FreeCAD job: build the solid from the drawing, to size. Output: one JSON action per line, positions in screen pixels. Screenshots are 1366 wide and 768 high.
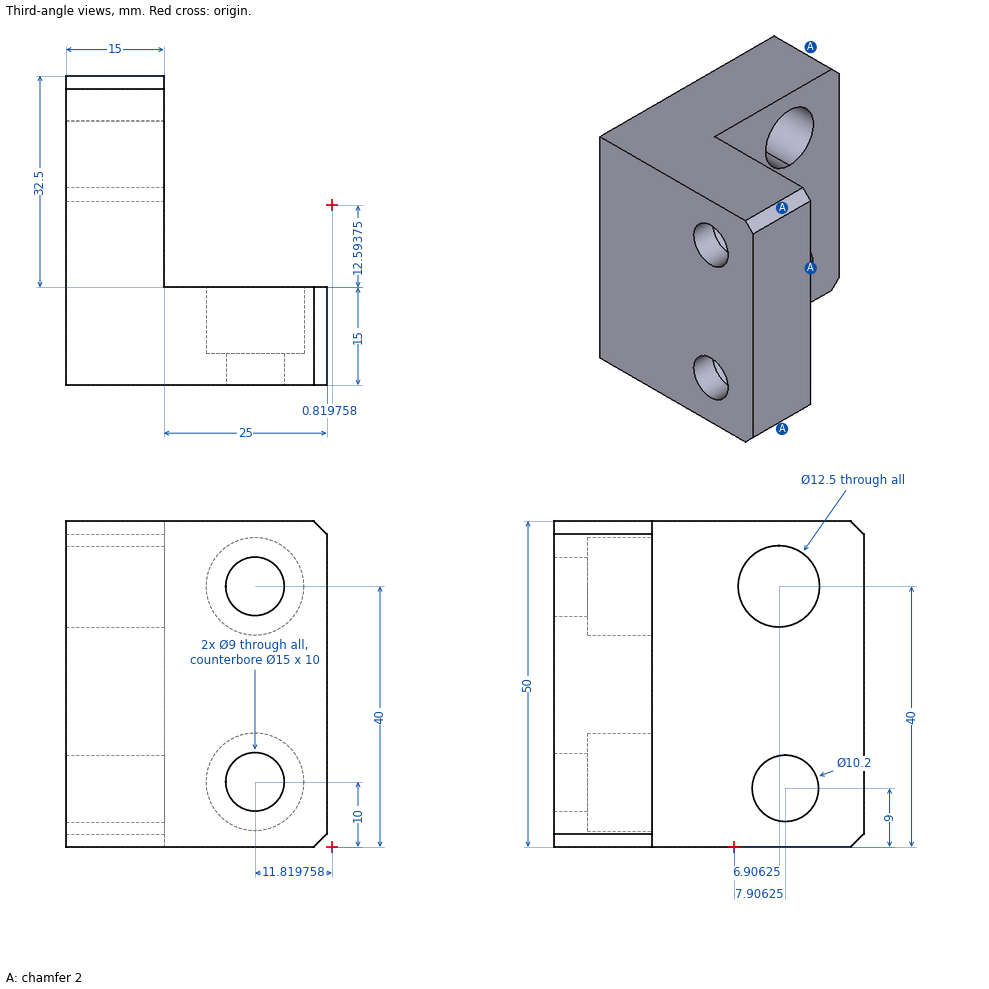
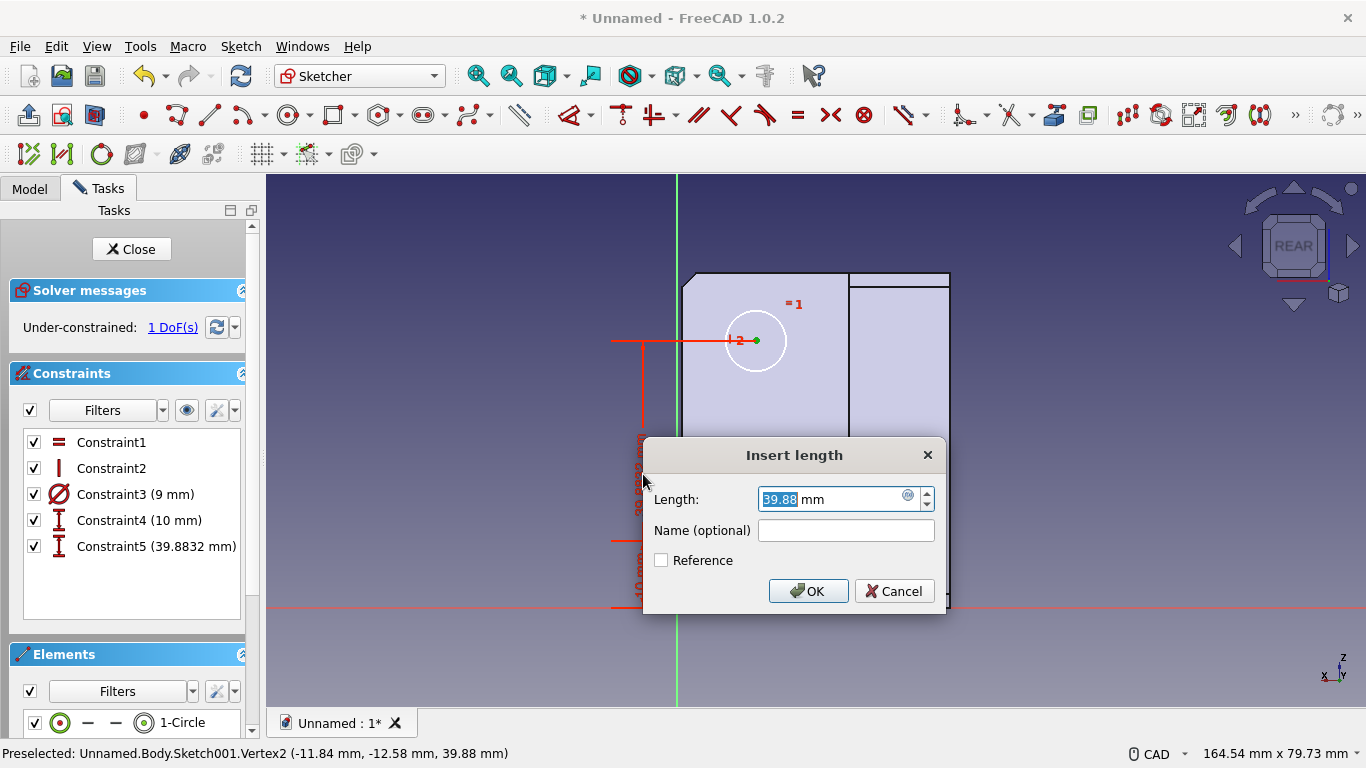
{"action": "type", "text": "40"}
{"action": "key", "text": "Return"}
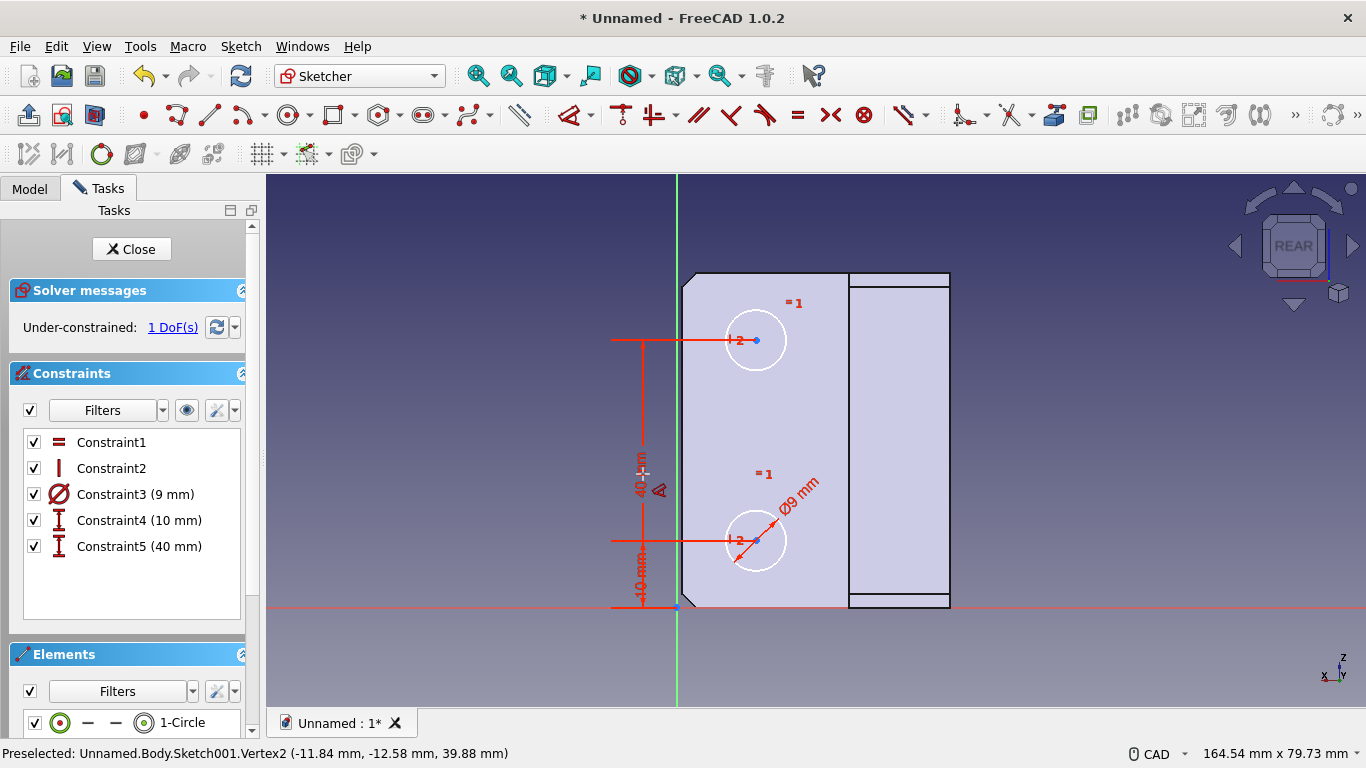
{"action": "left_click", "coordinate": [756, 541]}
{"action": "left_click", "coordinate": [716, 642]}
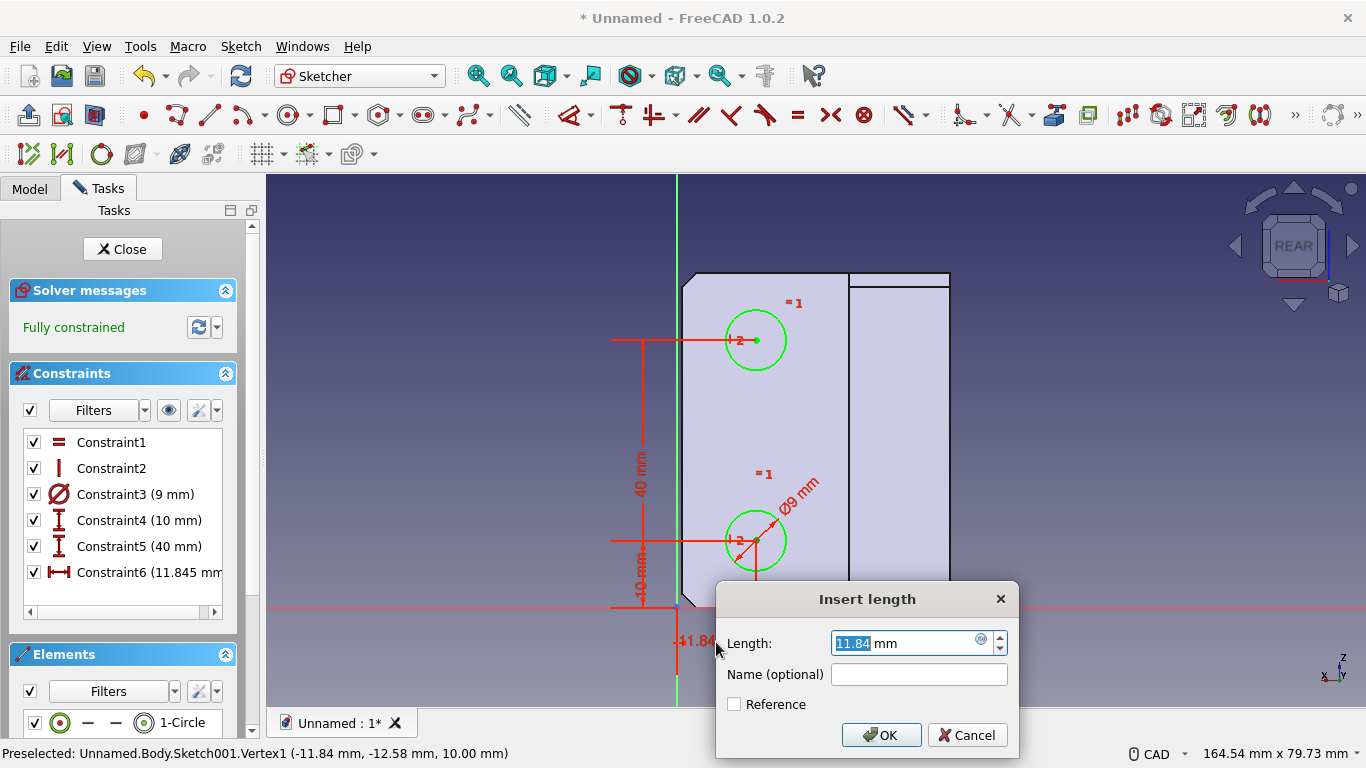
{"action": "type", "text": "11.819758"}
{"action": "key", "text": "Return"}
{"action": "key", "text": "Escape"}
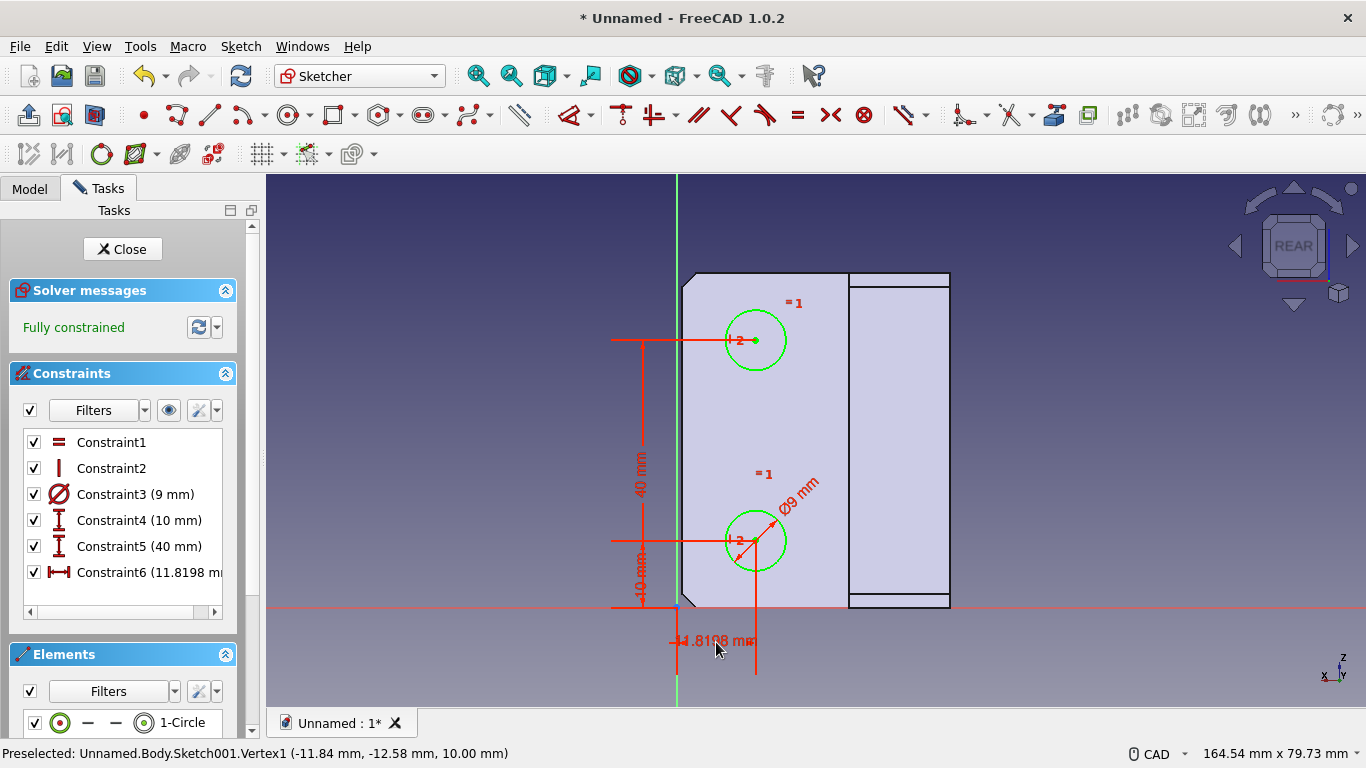
{"action": "left_click", "coordinate": [123, 249]}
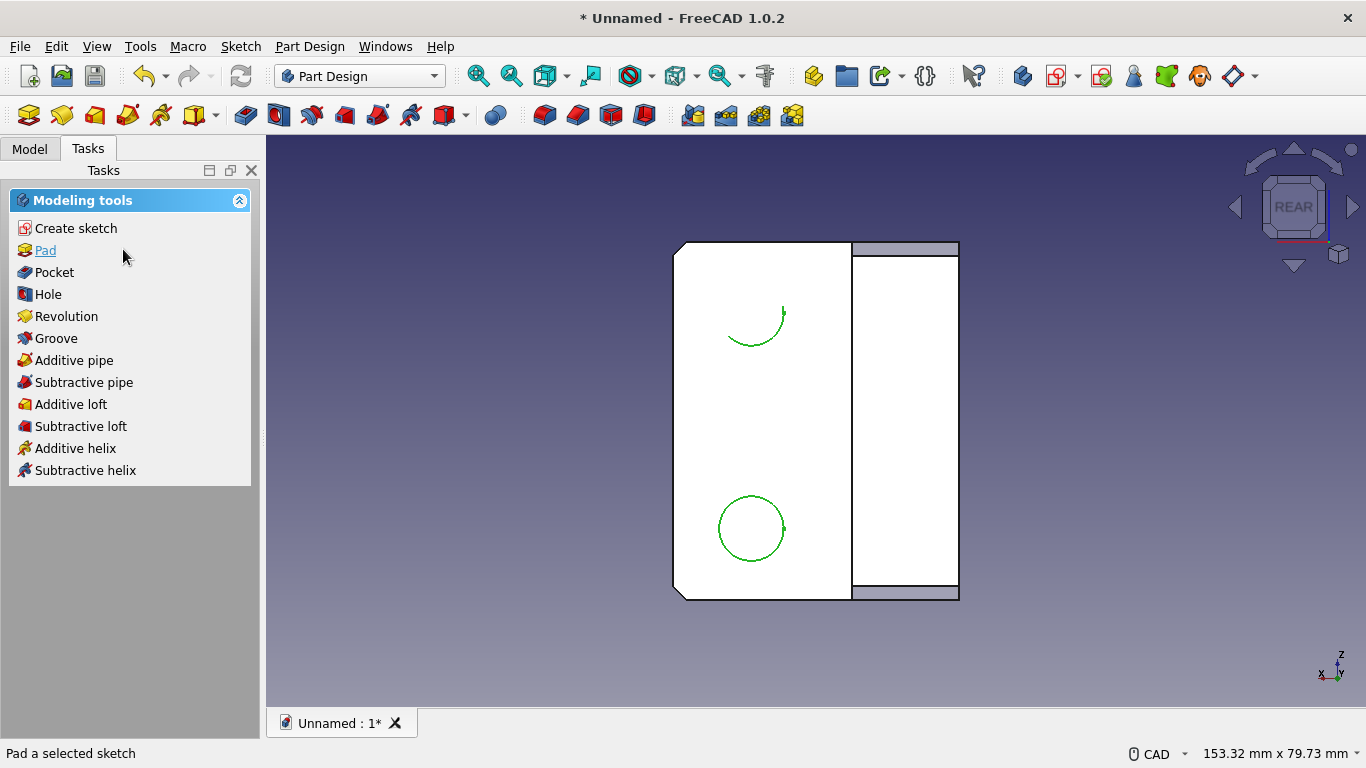
{"action": "left_click", "coordinate": [279, 116]}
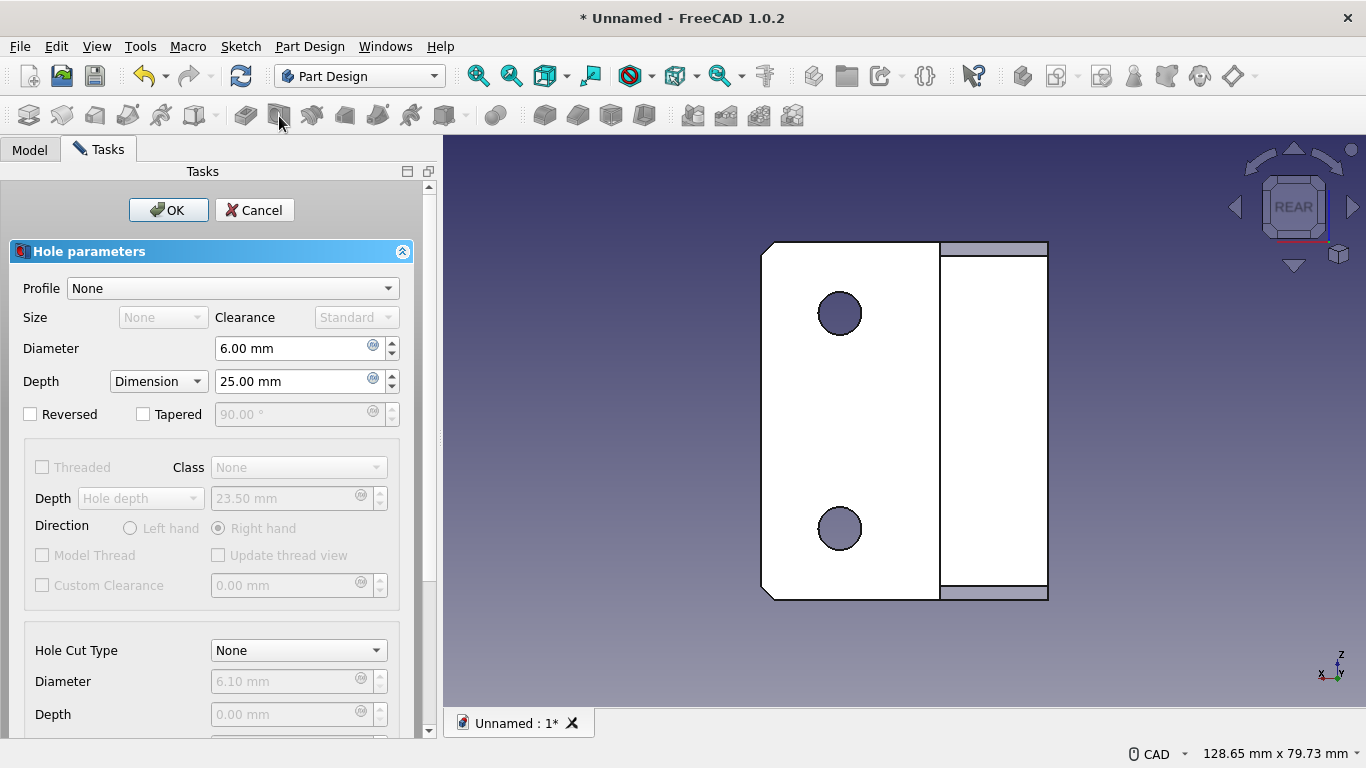
{"action": "triple_click", "coordinate": [300, 348]}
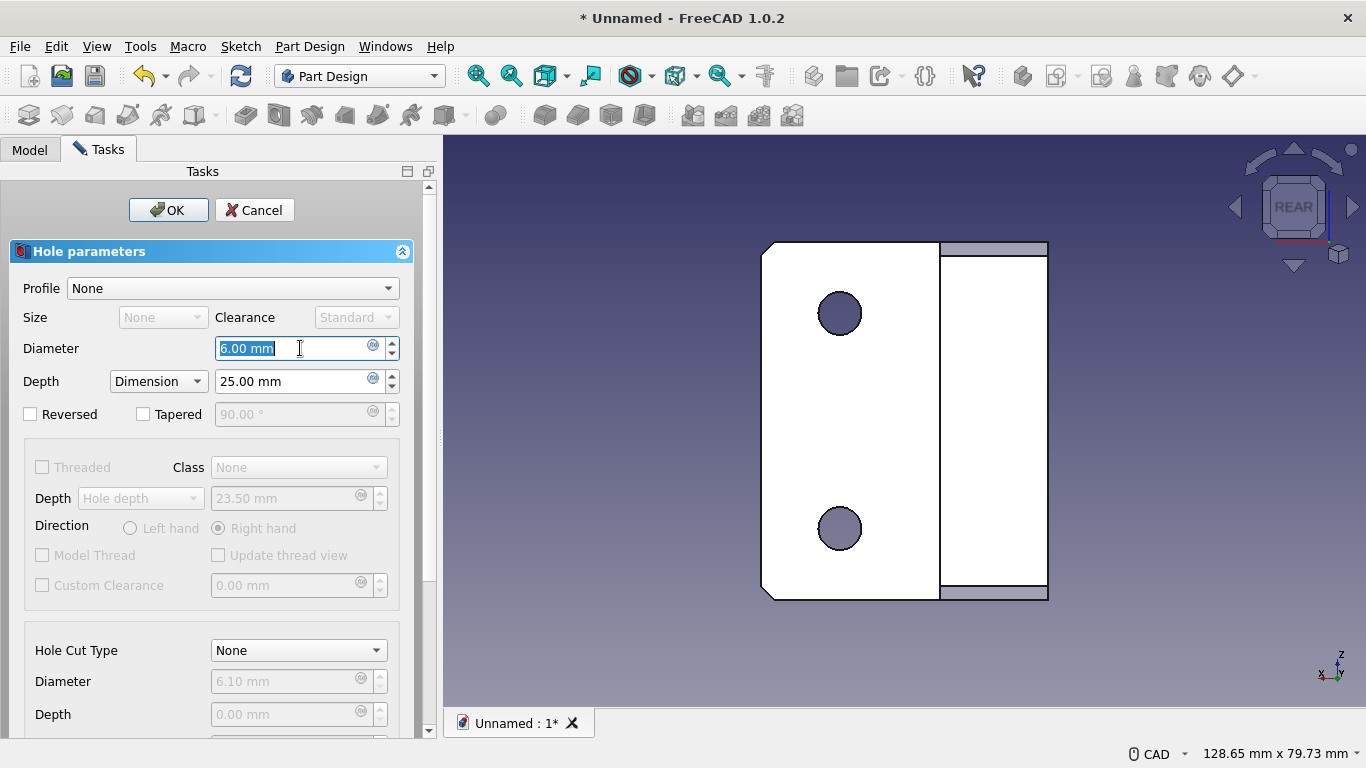
{"action": "type", "text": "9"}
{"action": "key", "text": "Tab"}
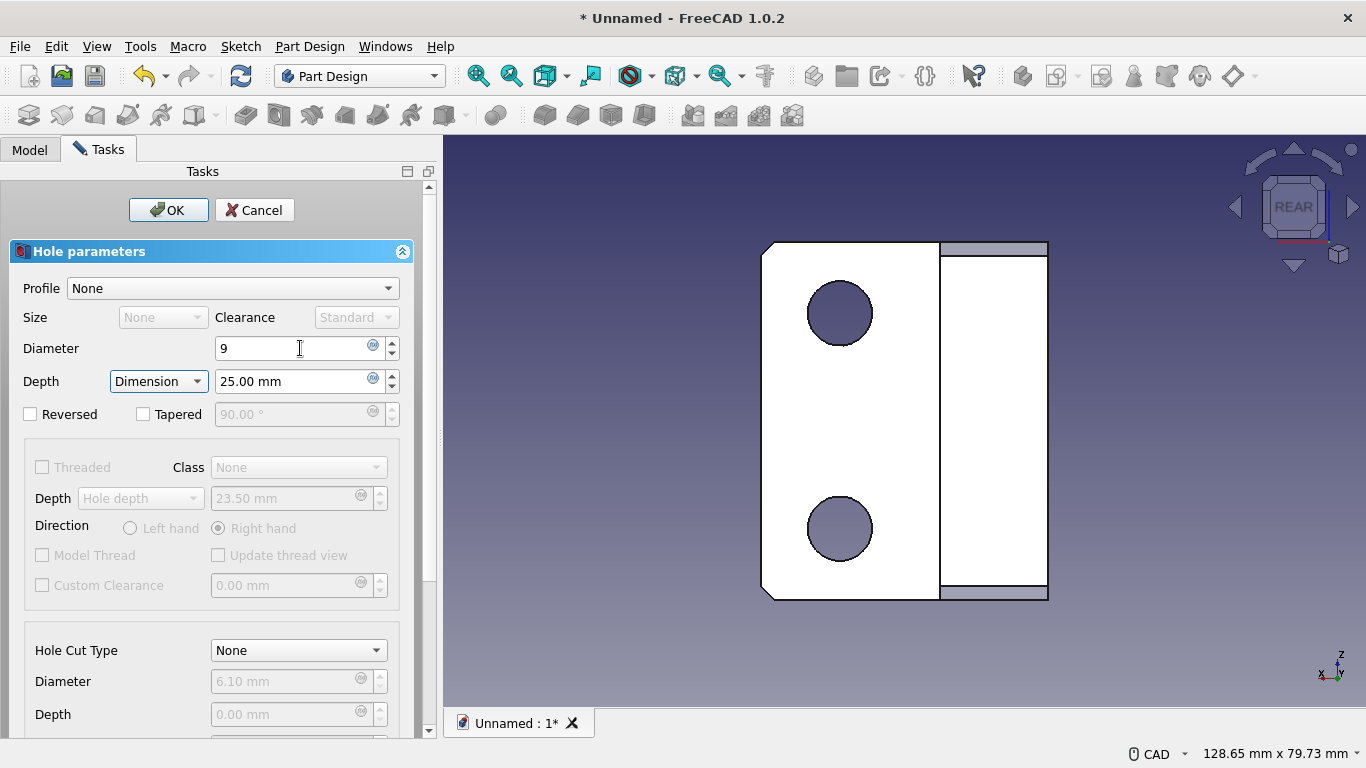
{"action": "left_click", "coordinate": [160, 382]}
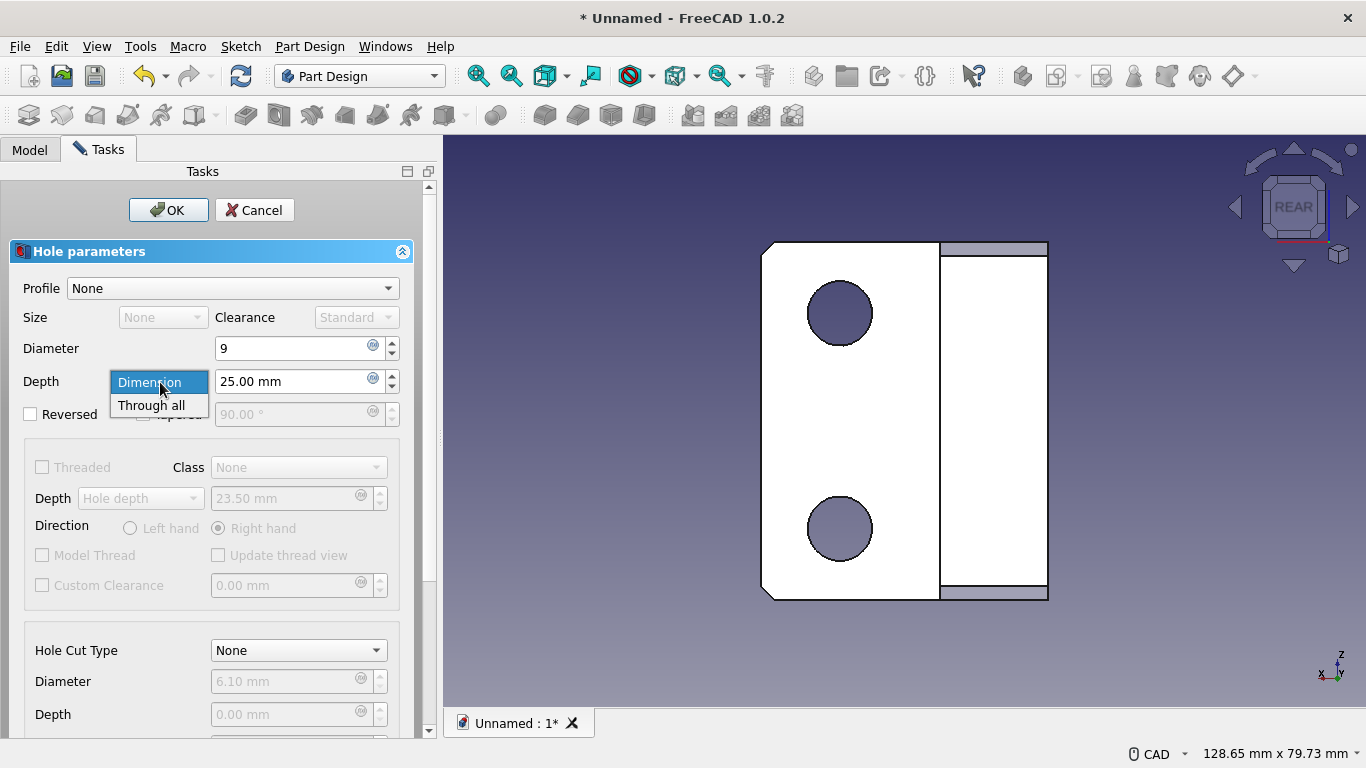
{"action": "left_click", "coordinate": [158, 406]}